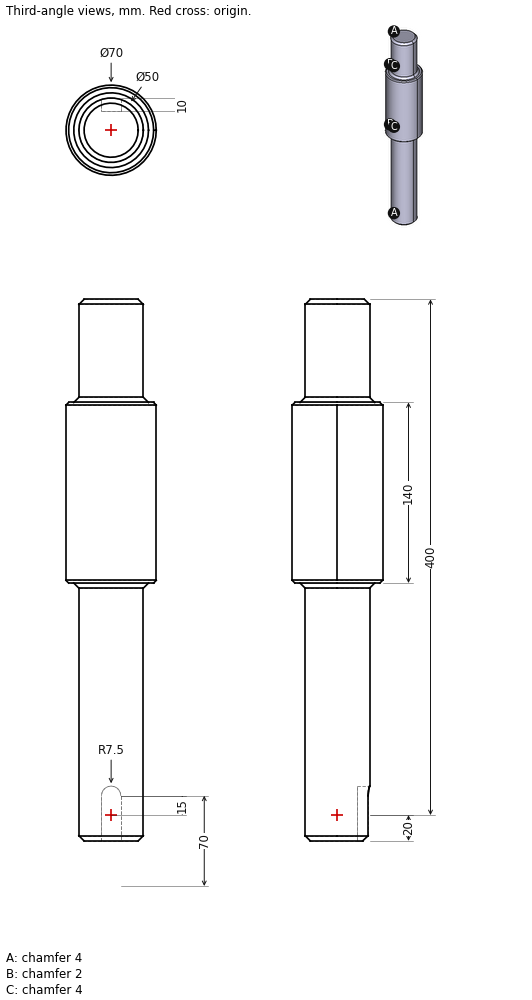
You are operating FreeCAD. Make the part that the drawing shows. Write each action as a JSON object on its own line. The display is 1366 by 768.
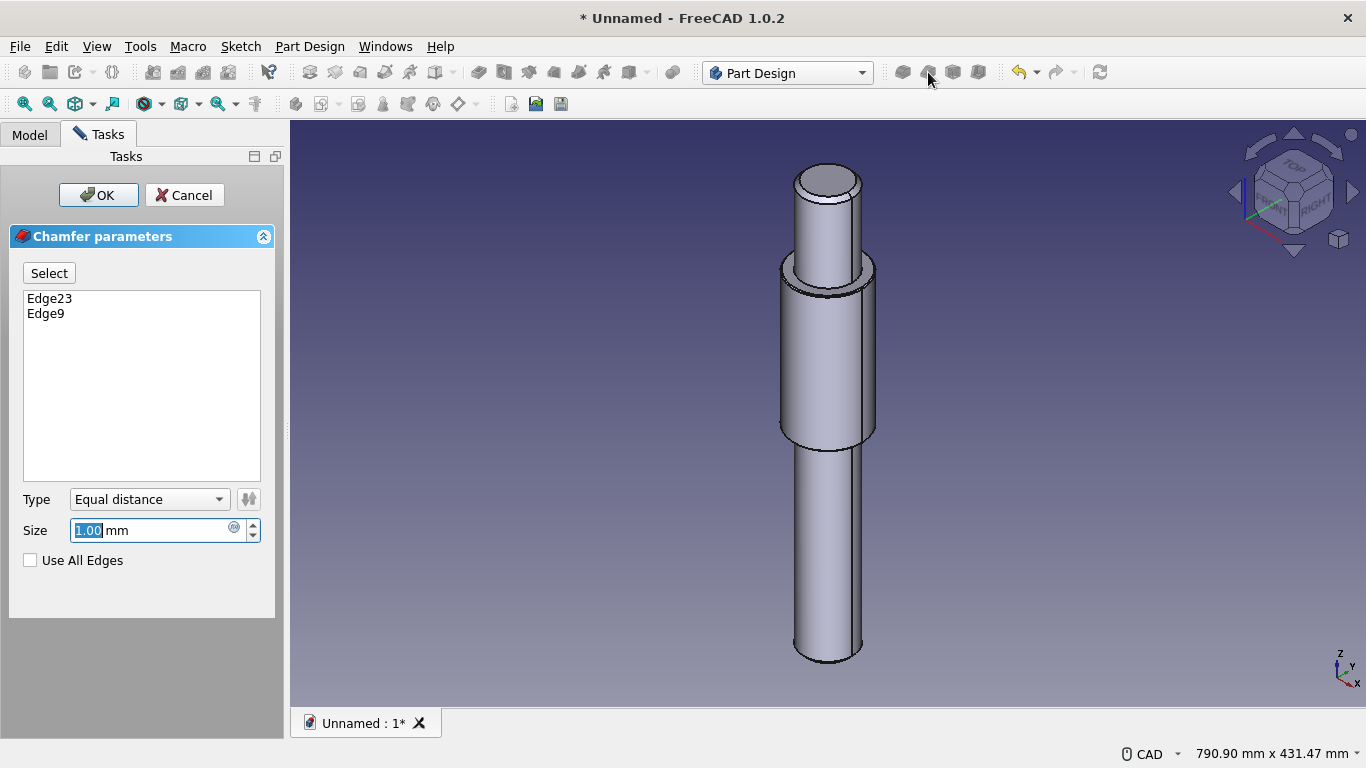
{"action": "type", "text": "2"}
{"action": "key", "text": "Tab"}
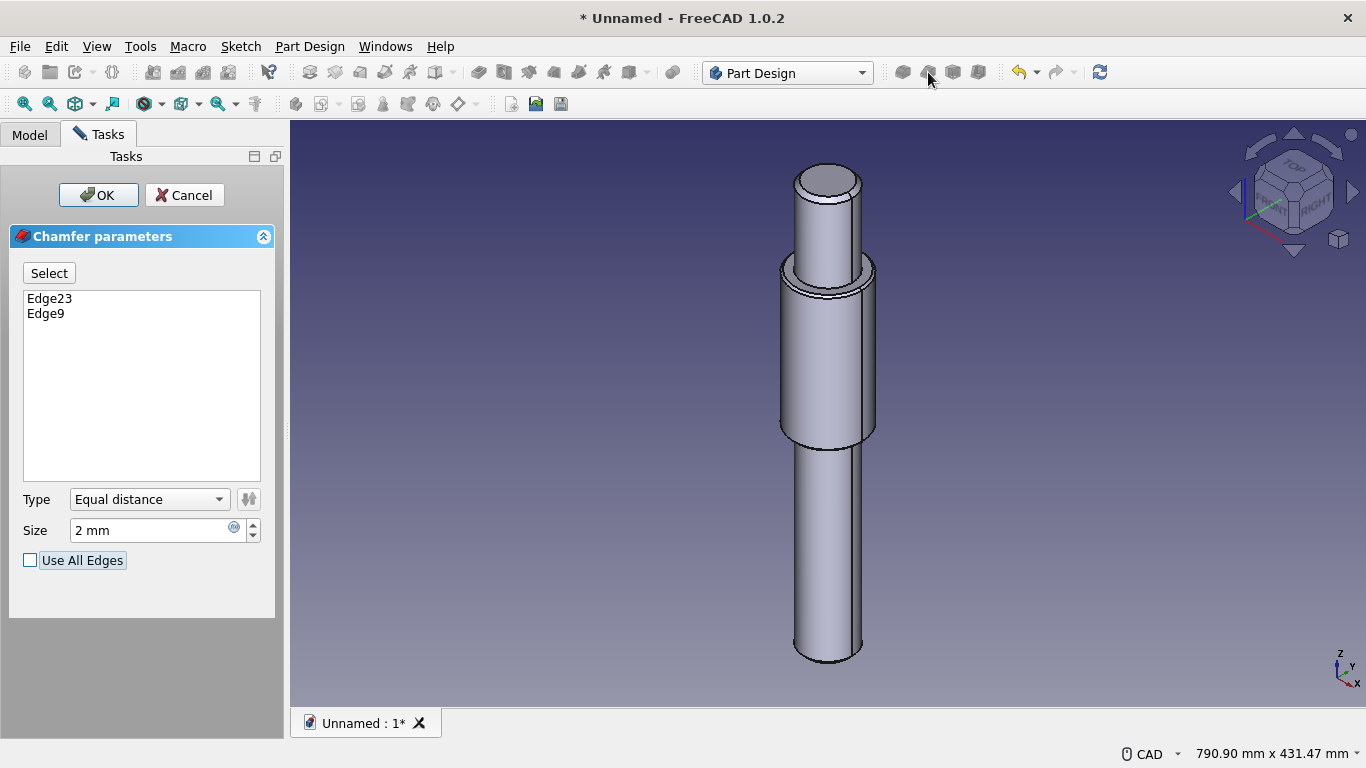
{"action": "left_click", "coordinate": [99, 195]}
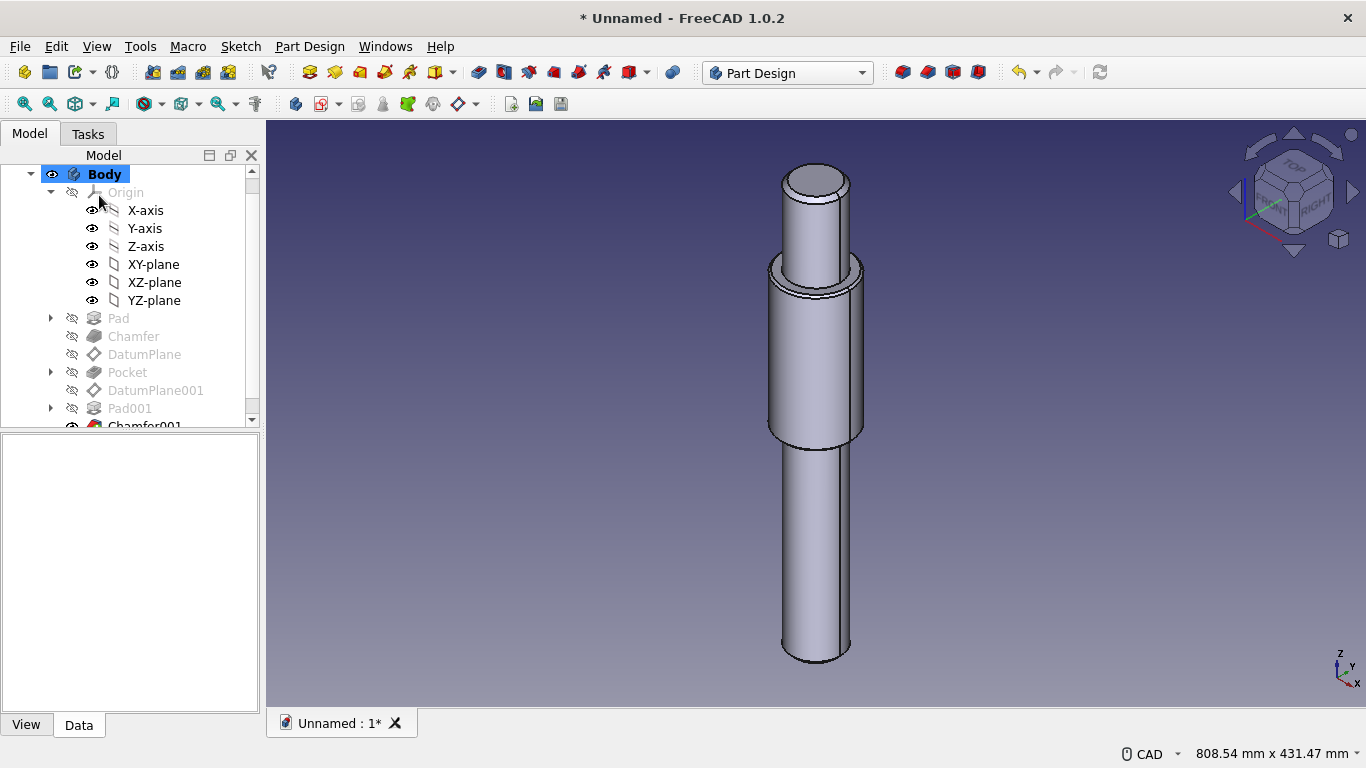
{"action": "key", "text": "2"}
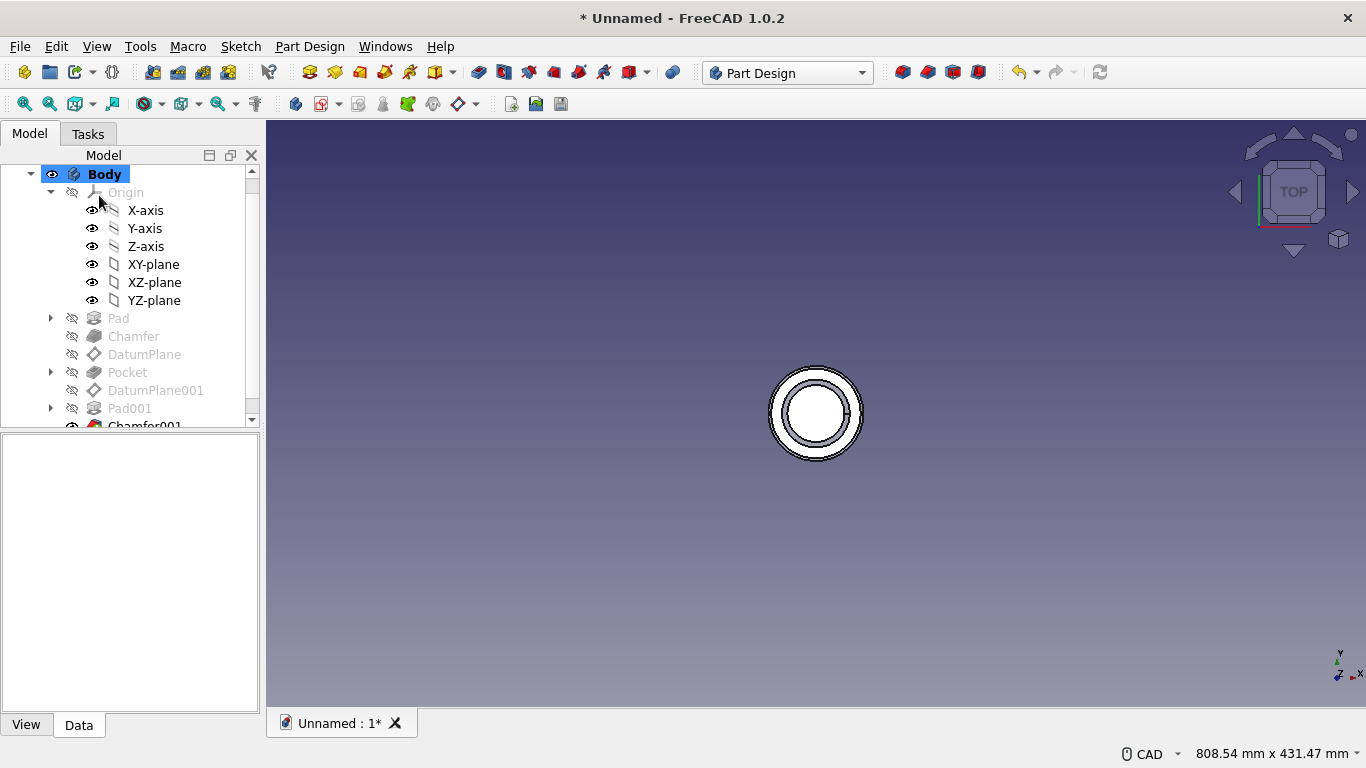
{"action": "left_click", "coordinate": [25, 104]}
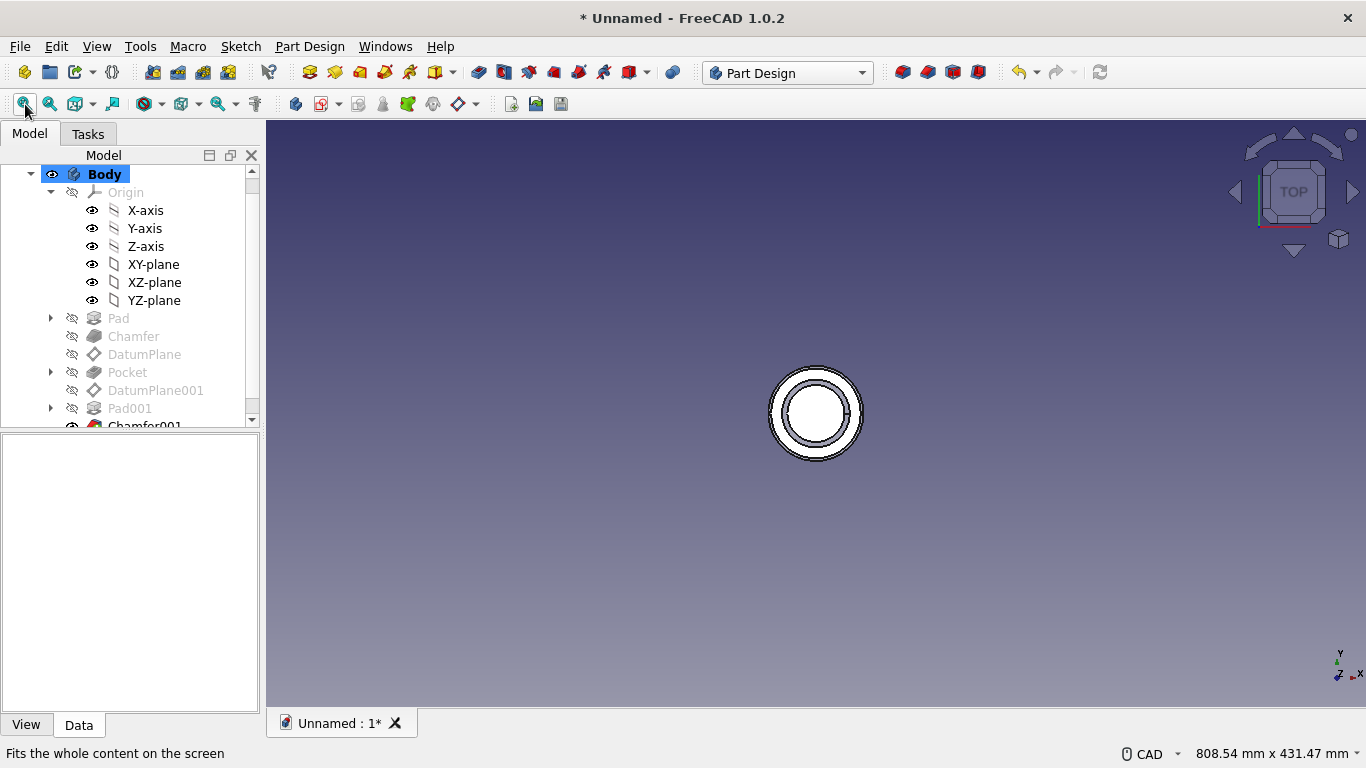
{"action": "key", "text": "0"}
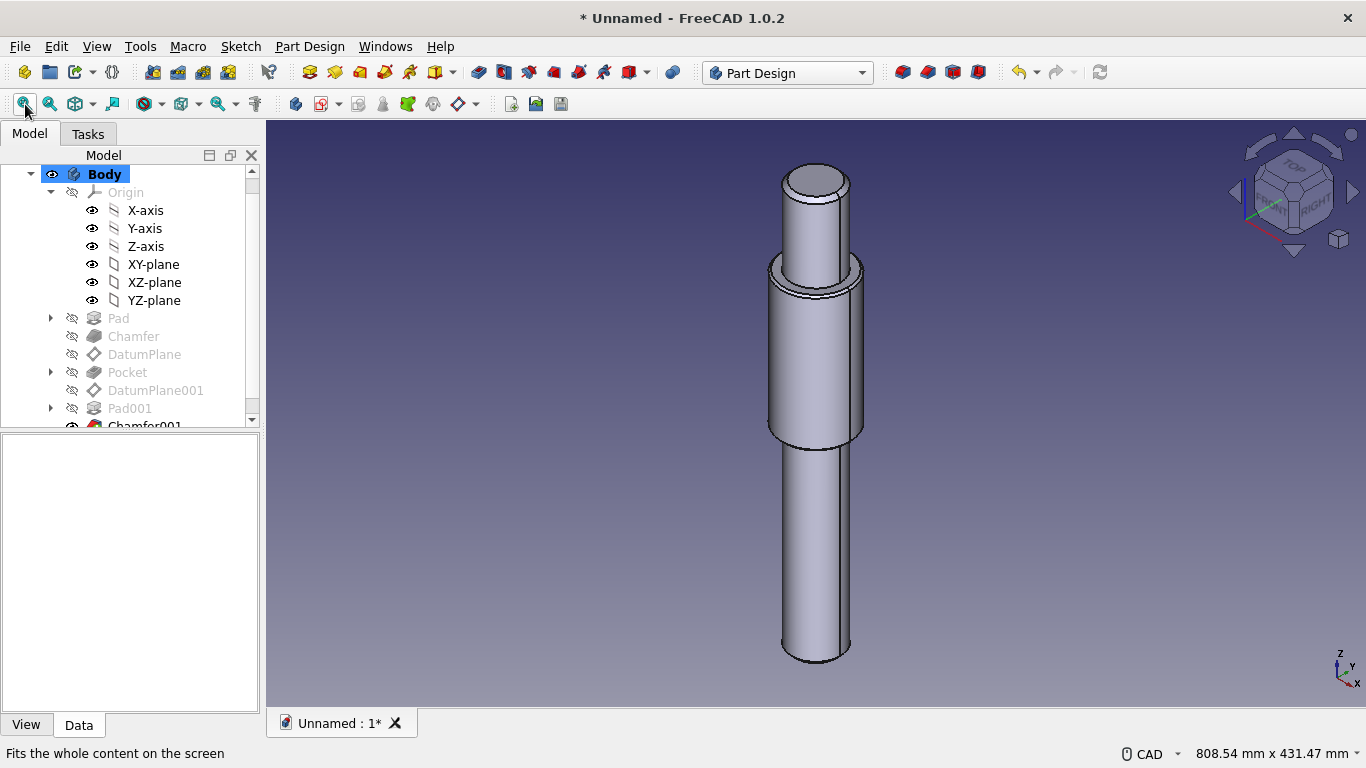
{"action": "key", "text": "1"}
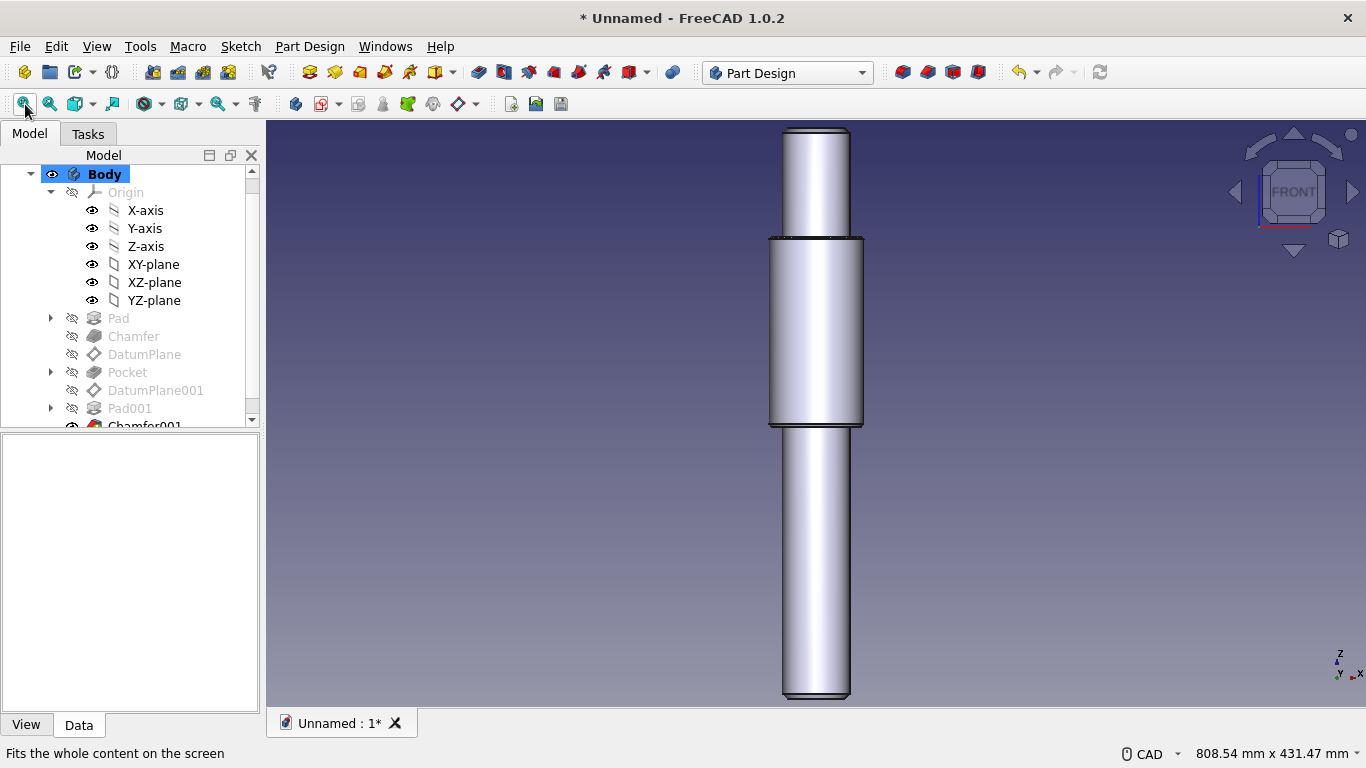
{"action": "key", "text": "3"}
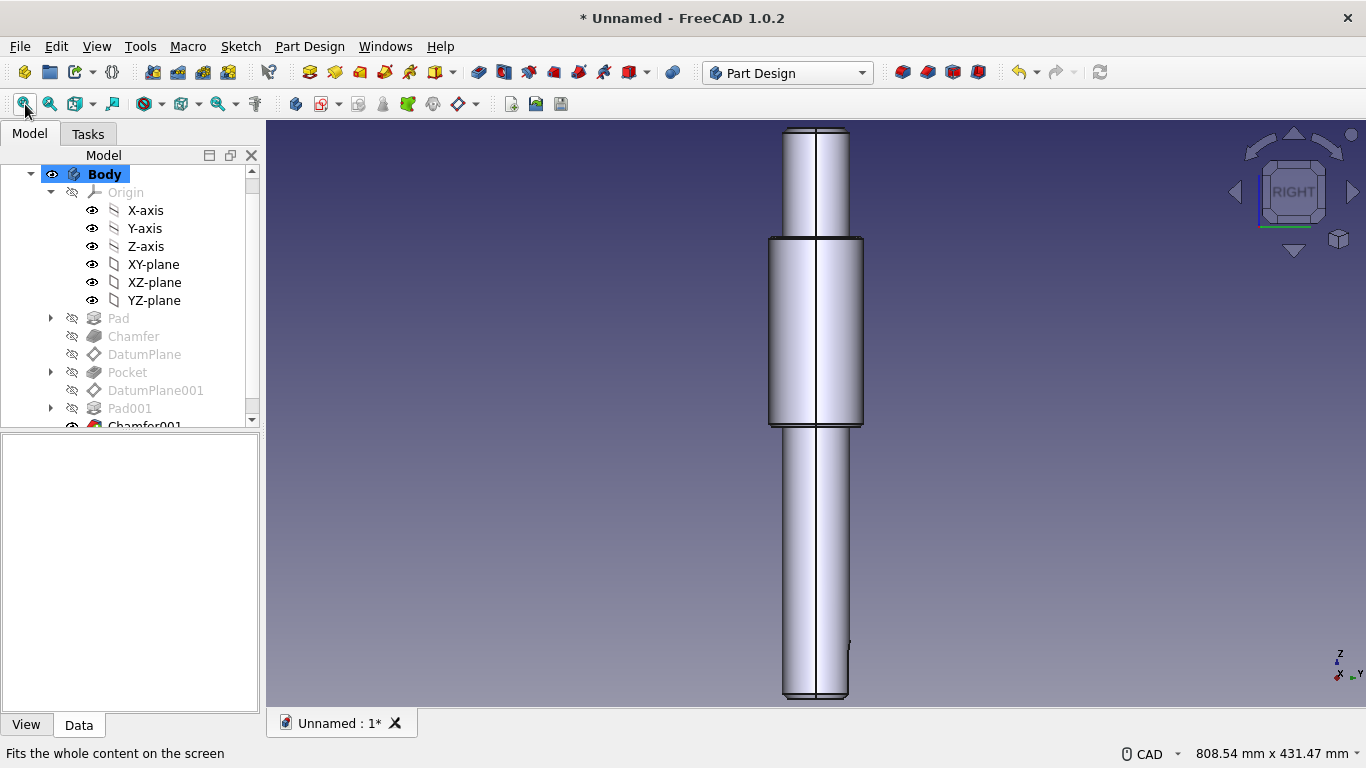
{"action": "key", "text": "5"}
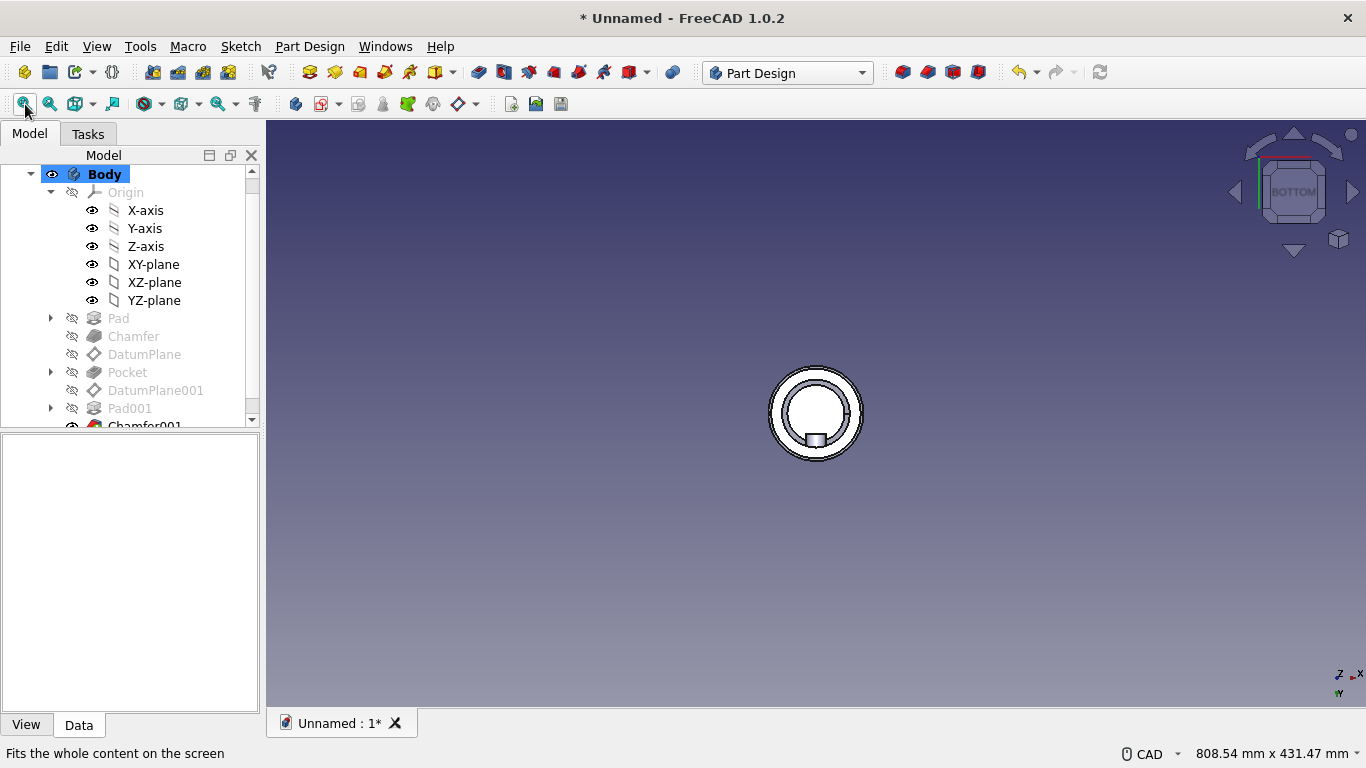
{"action": "left_click", "coordinate": [25, 104]}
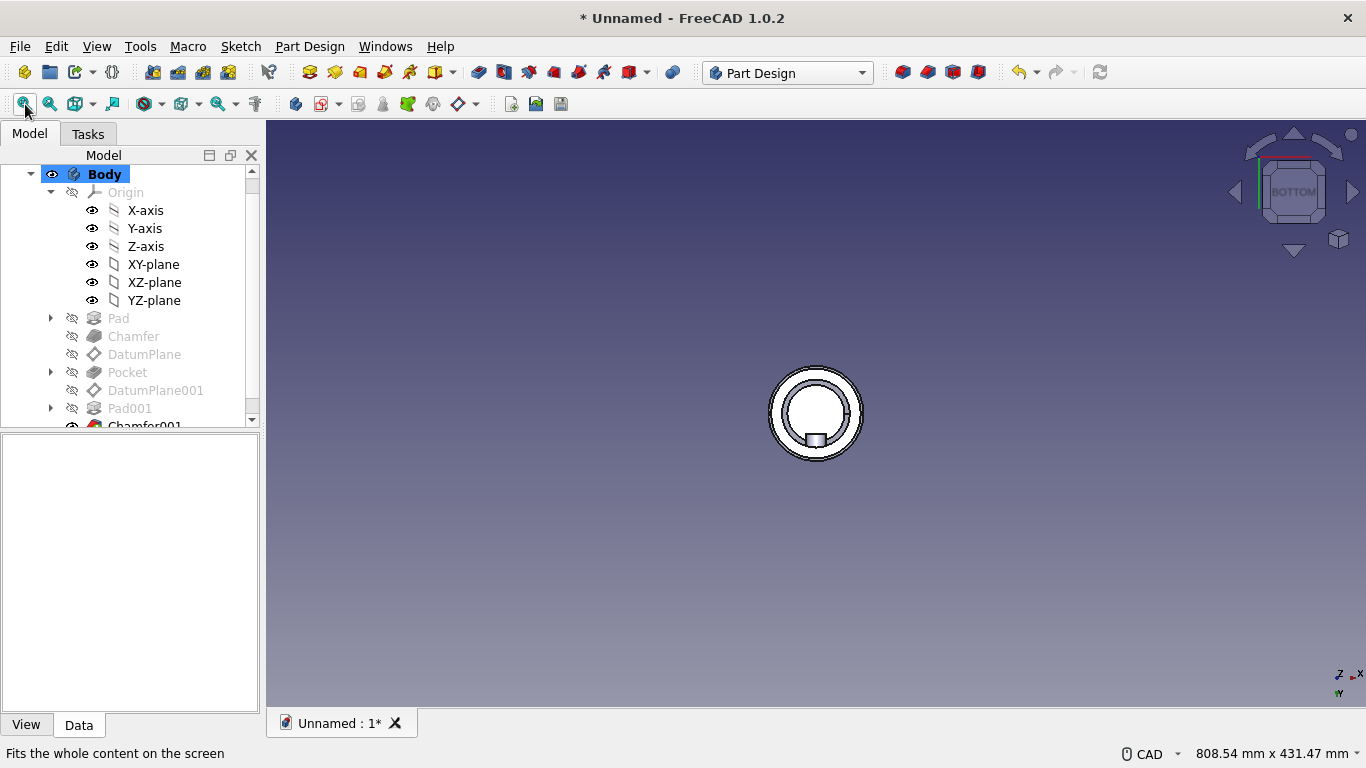
{"action": "key", "text": "4"}